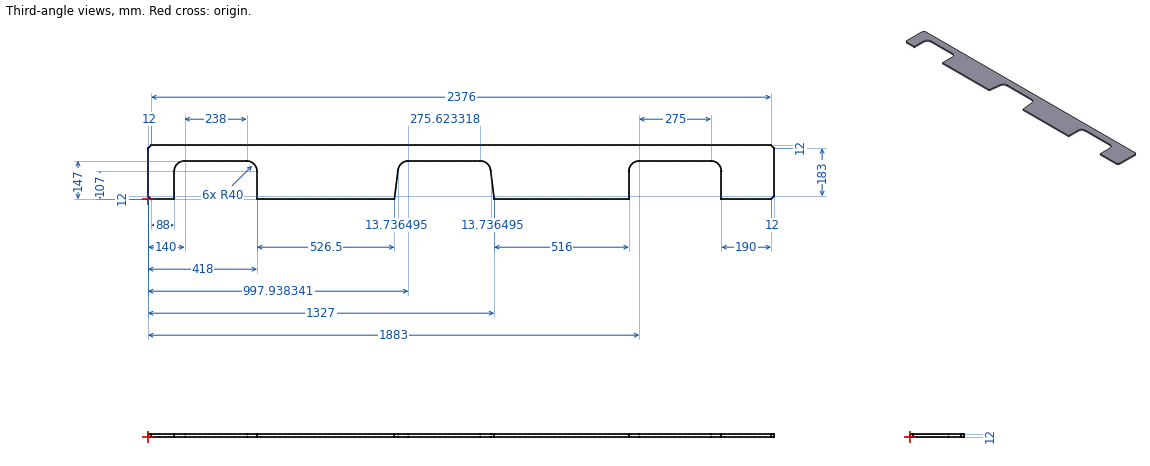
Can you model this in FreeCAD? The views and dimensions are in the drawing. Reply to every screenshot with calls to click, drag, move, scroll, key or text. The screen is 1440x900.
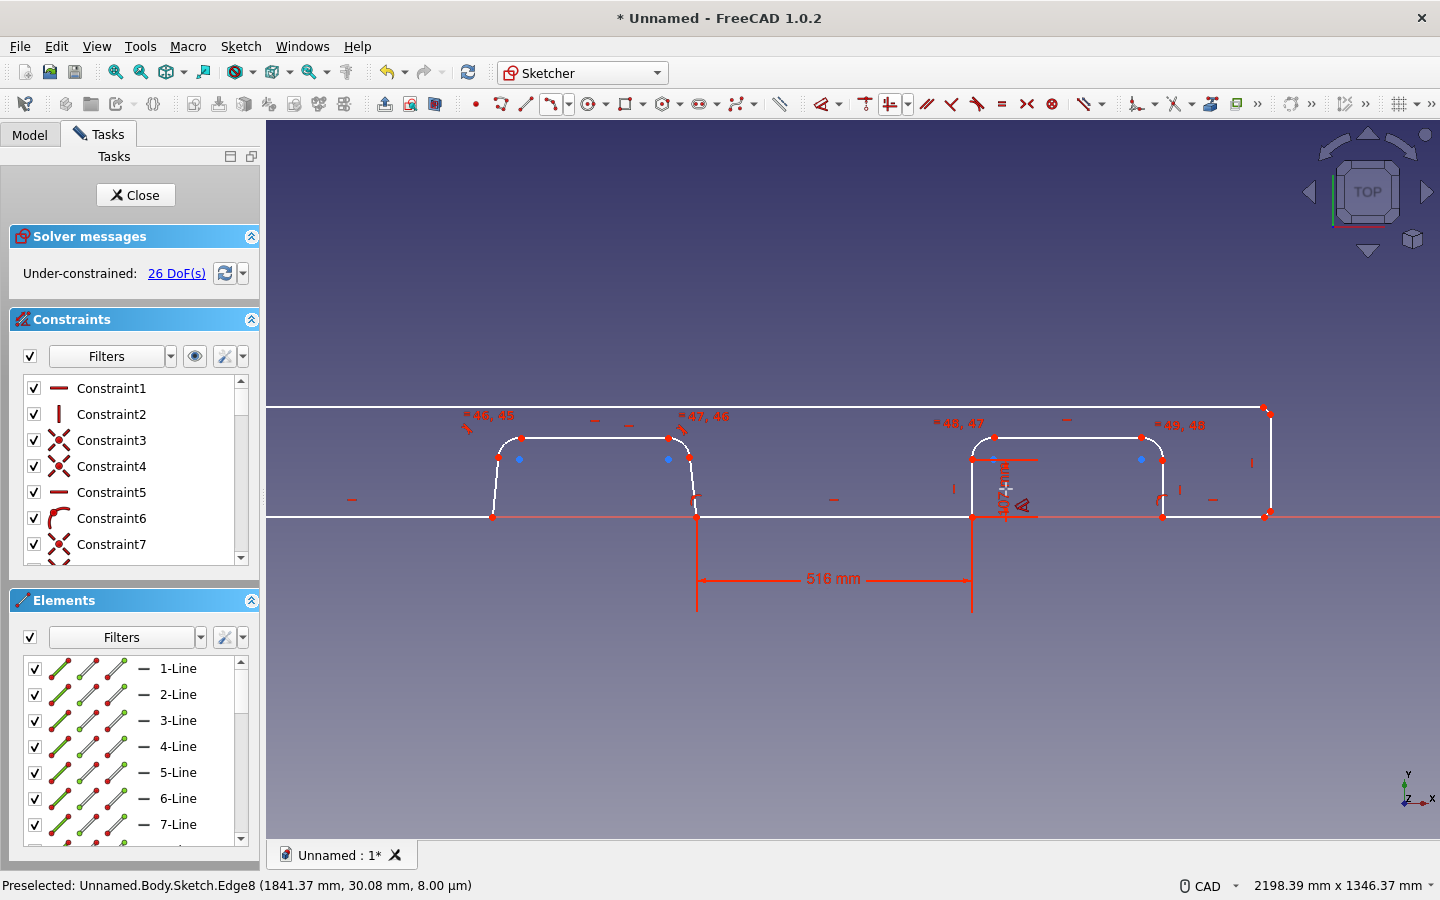
click(1038, 438)
click(1102, 472)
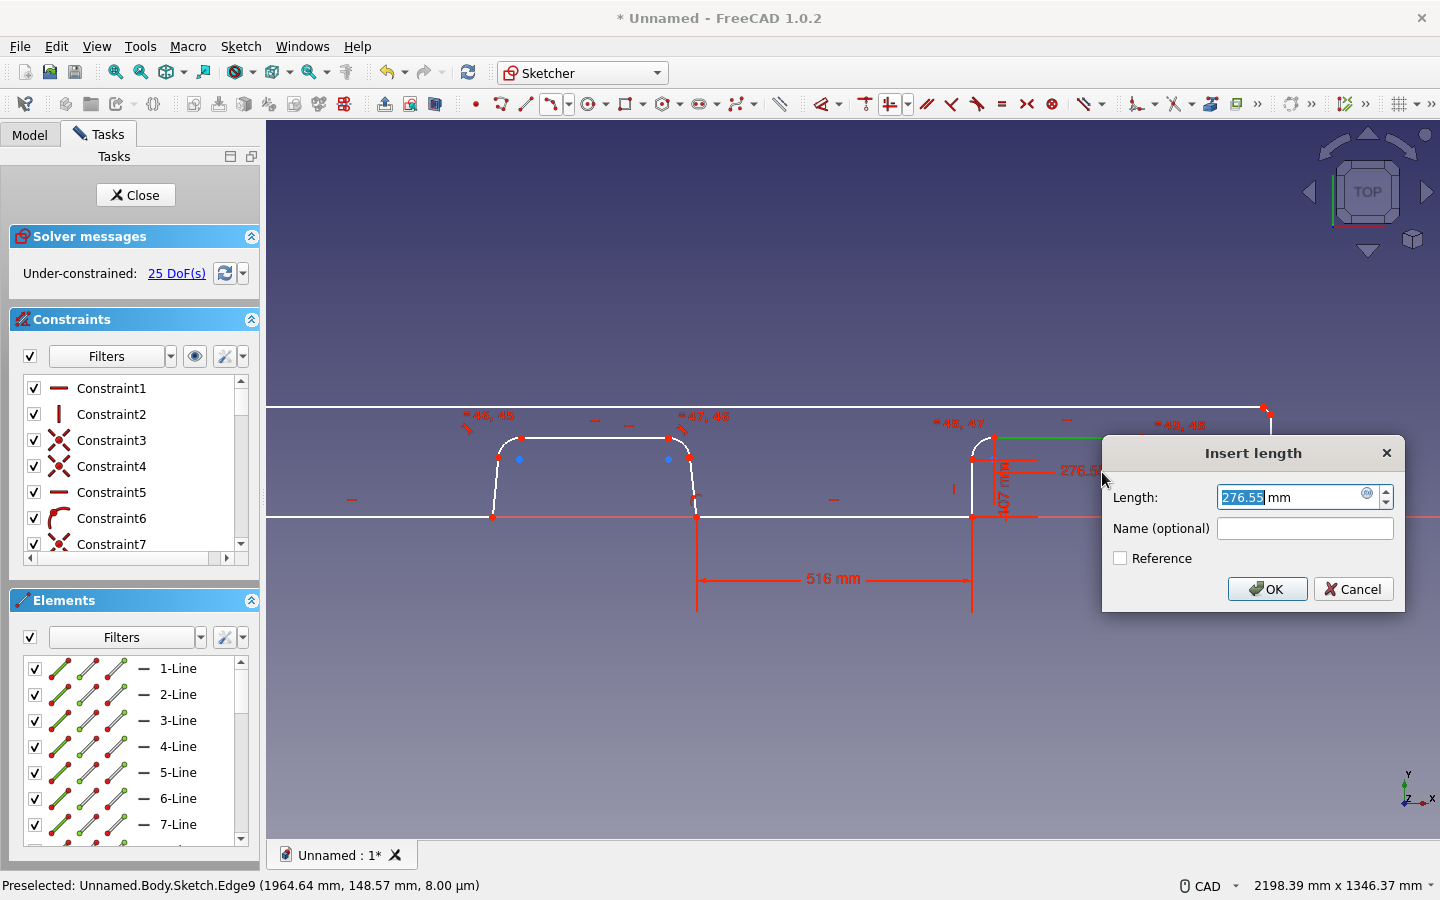
text(275)
key(Return)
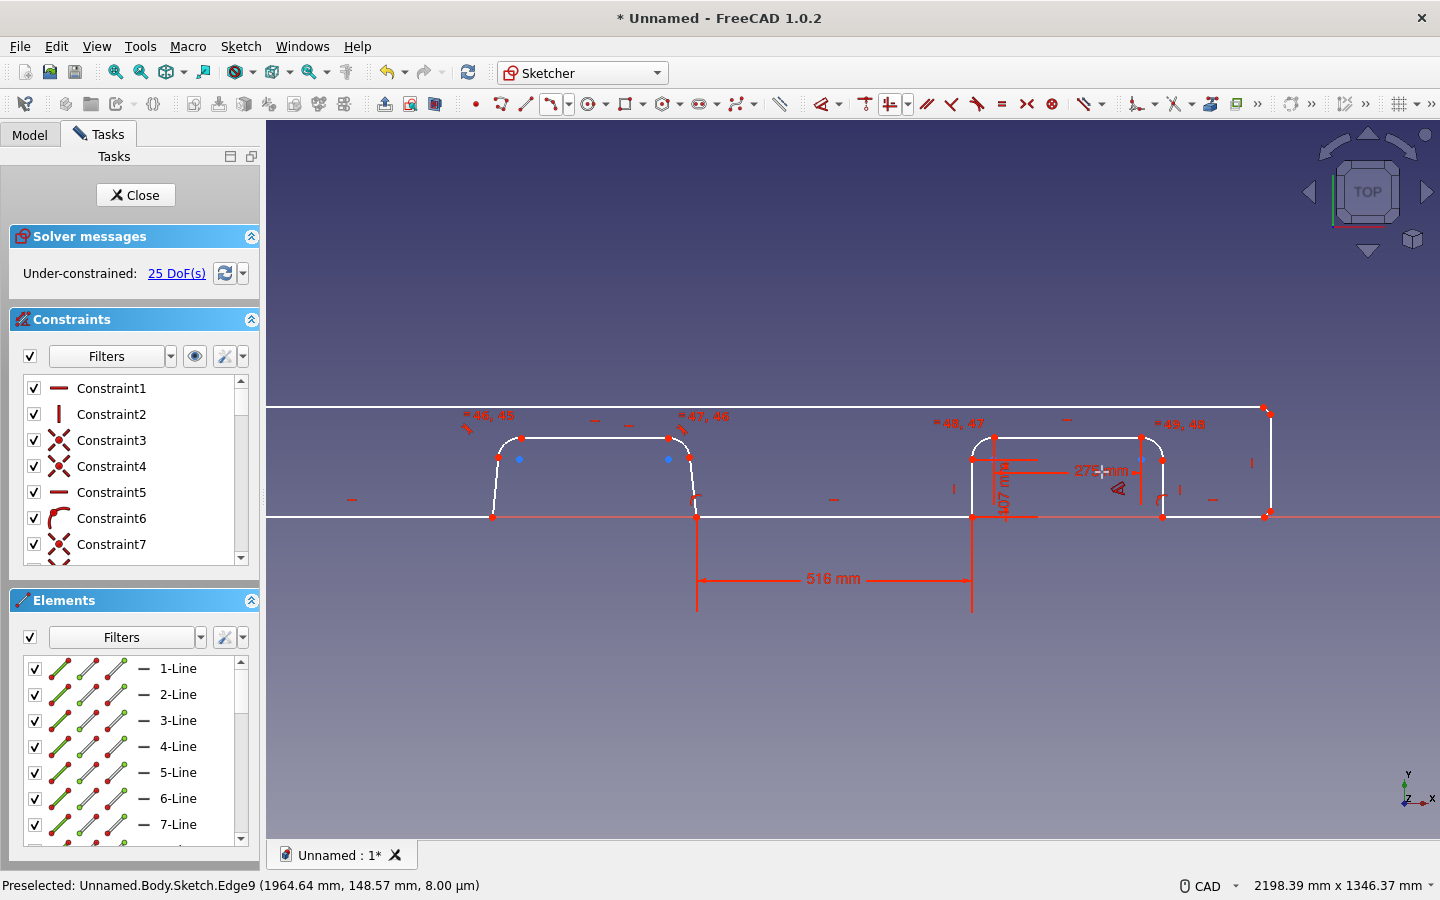
click(1163, 478)
click(1197, 489)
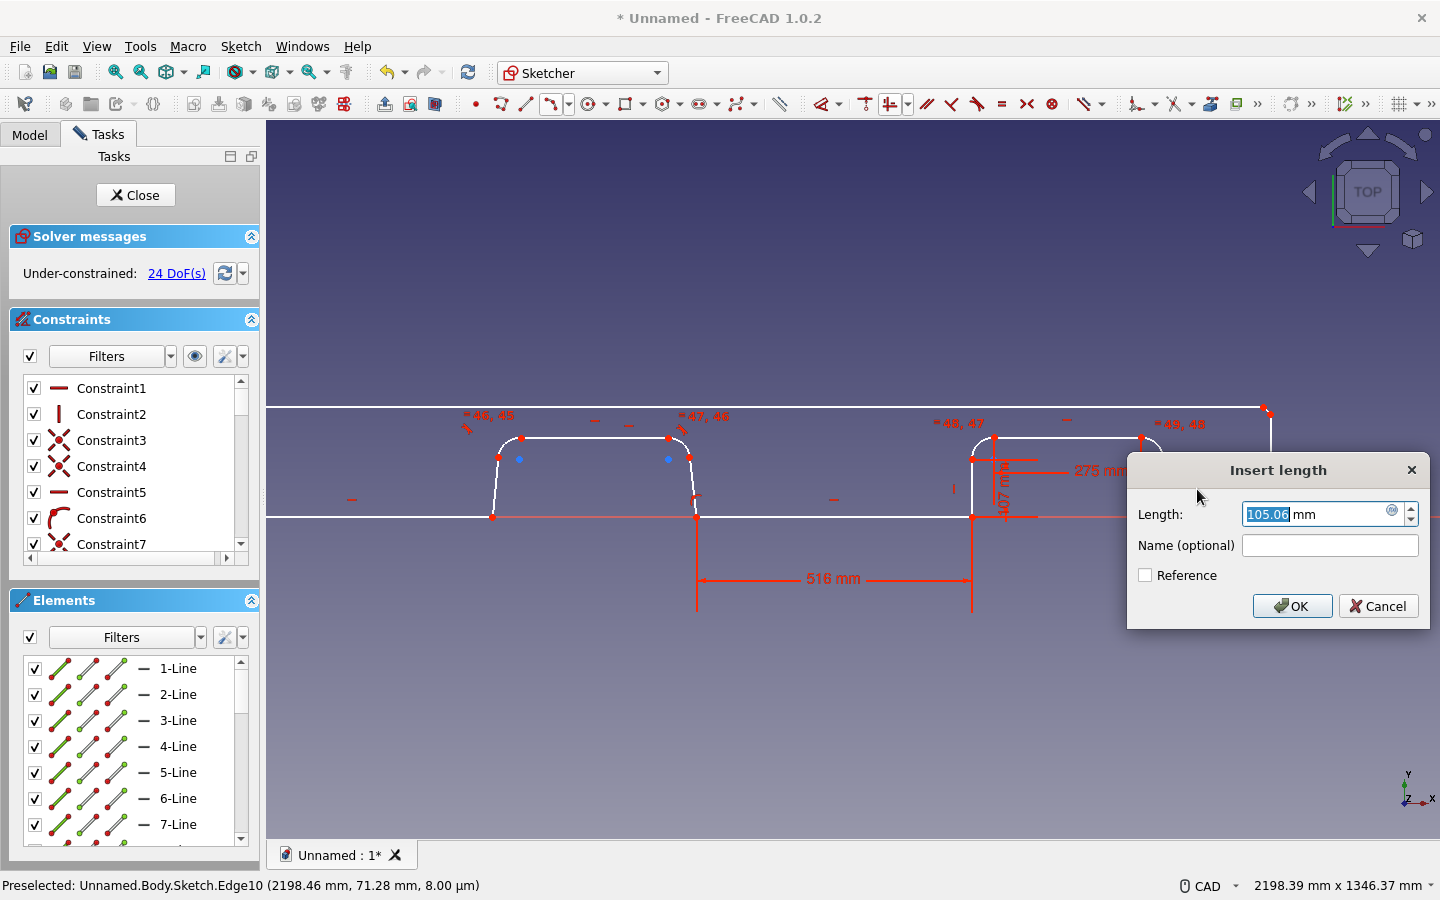
text(107)
key(Return)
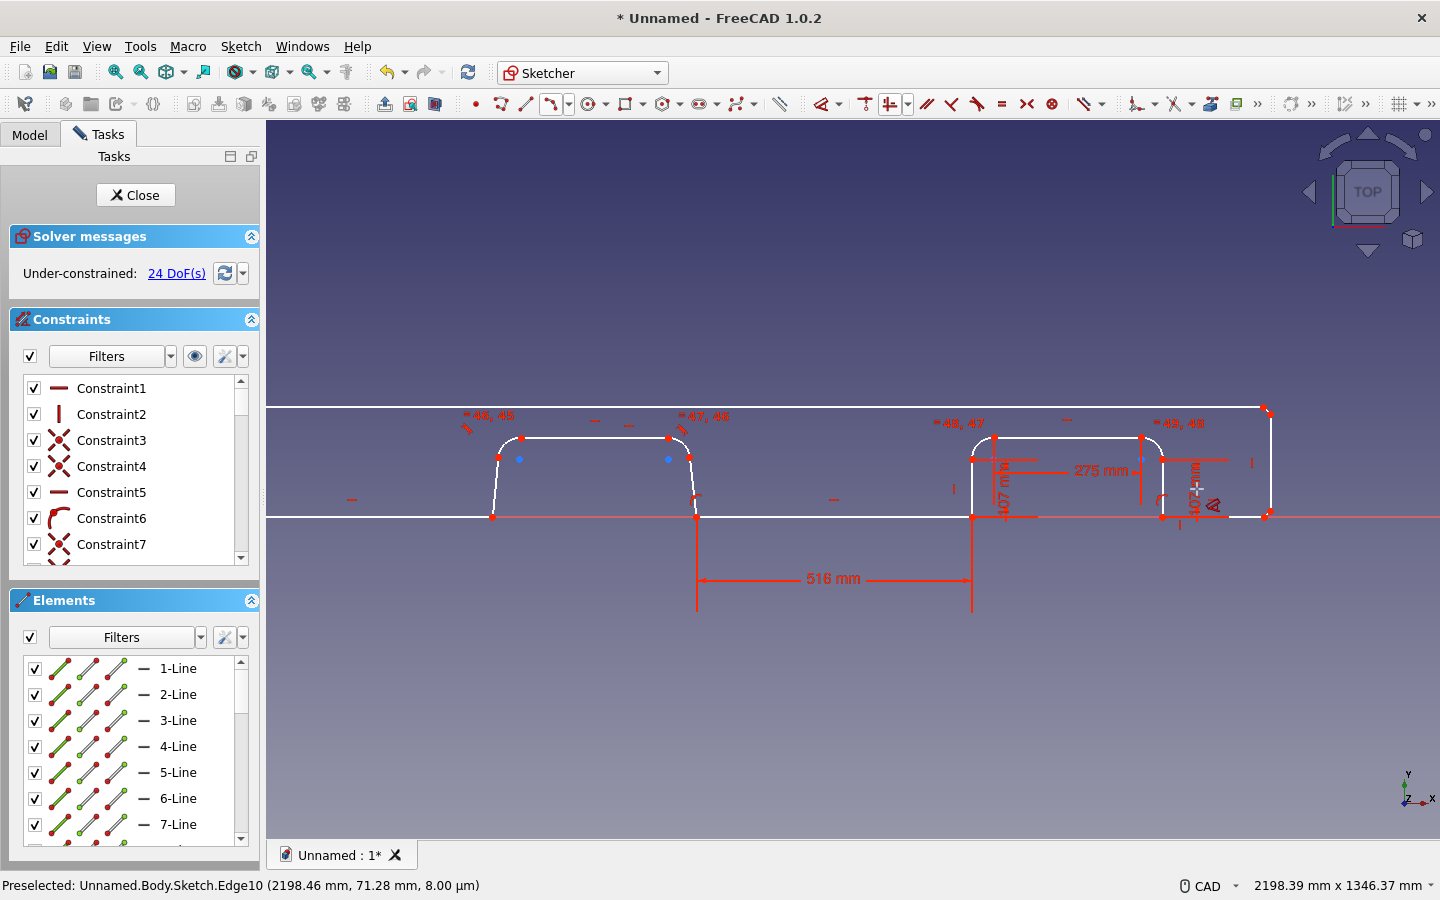
click(1193, 517)
click(1214, 551)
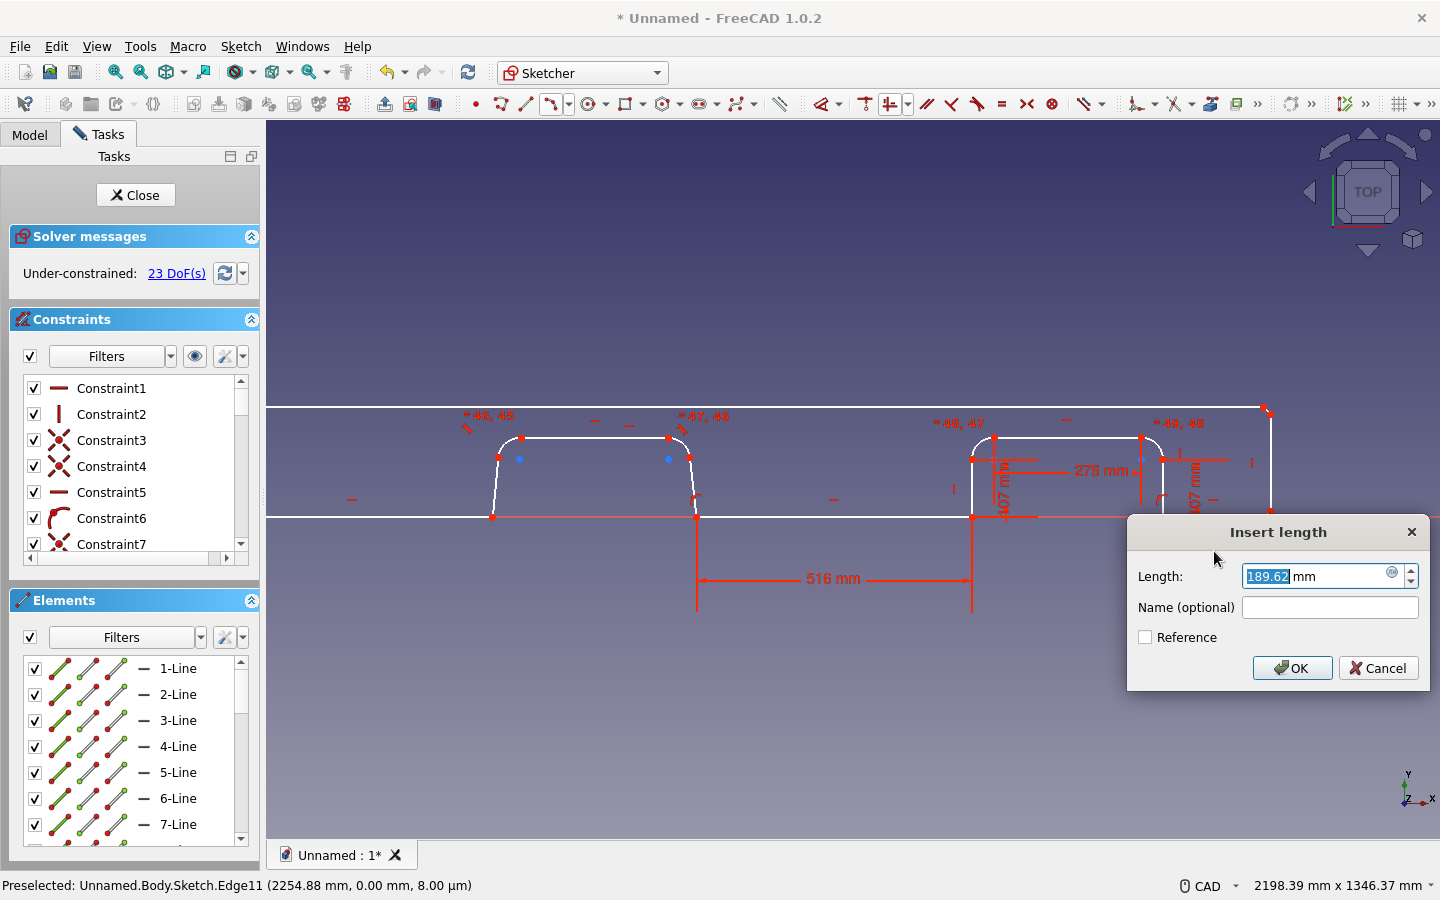
text(190)
key(Return)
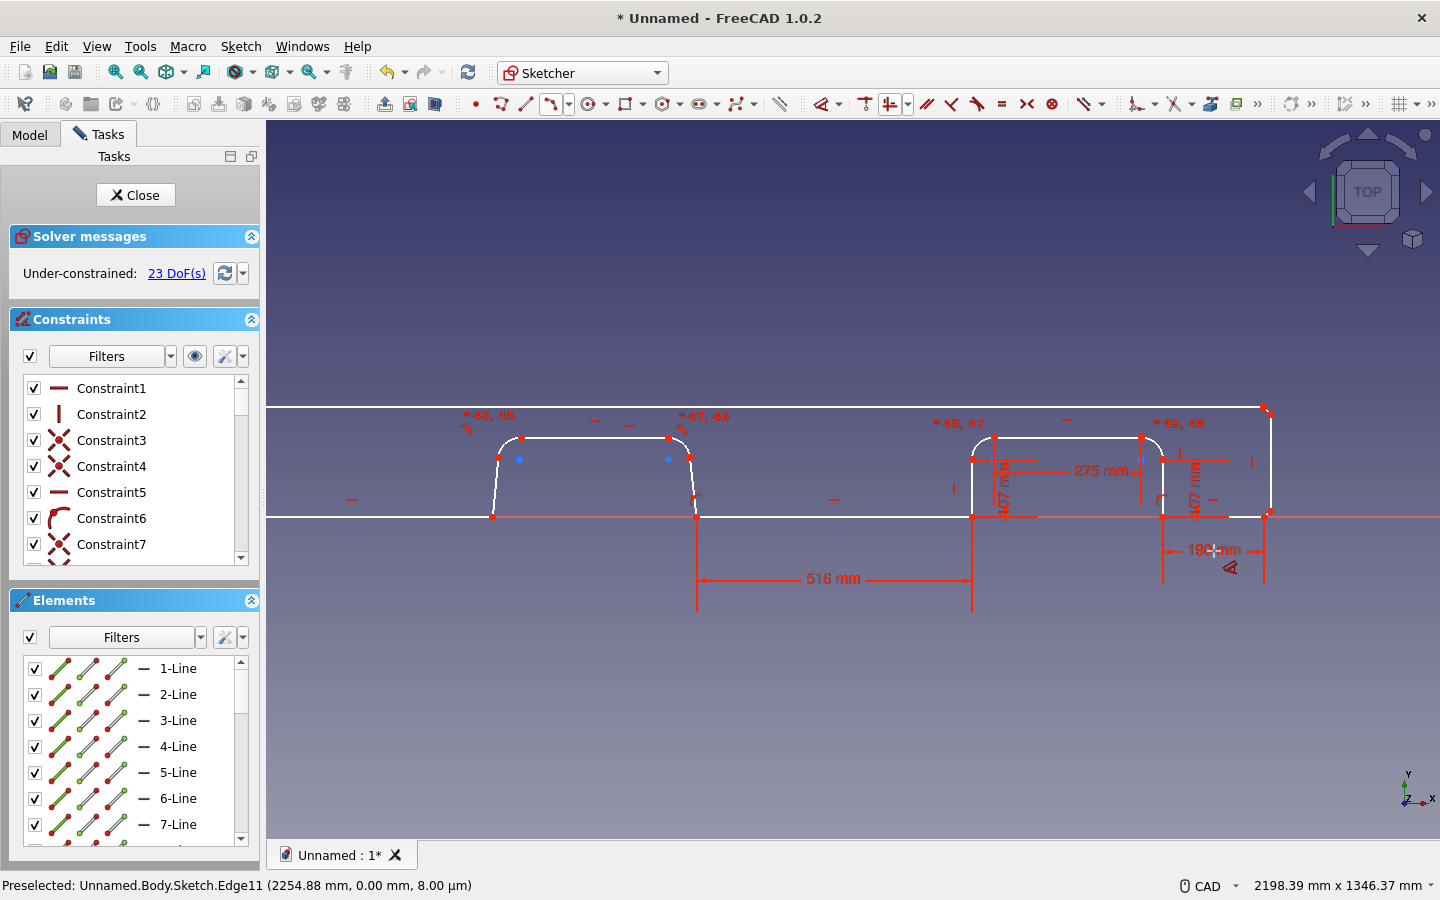
click(1271, 482)
click(1237, 463)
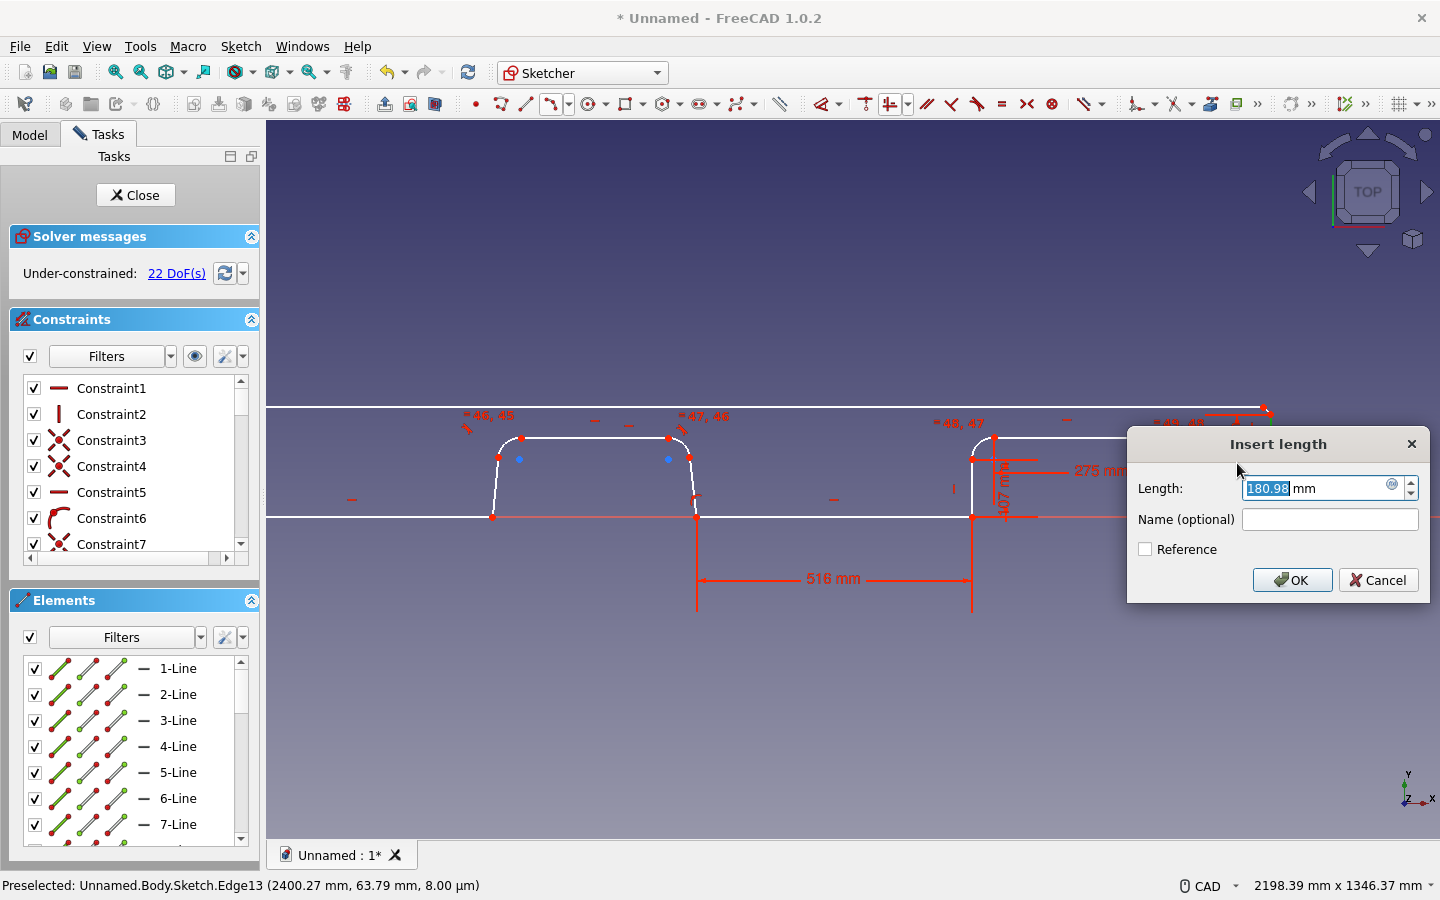
text(183)
key(Return)